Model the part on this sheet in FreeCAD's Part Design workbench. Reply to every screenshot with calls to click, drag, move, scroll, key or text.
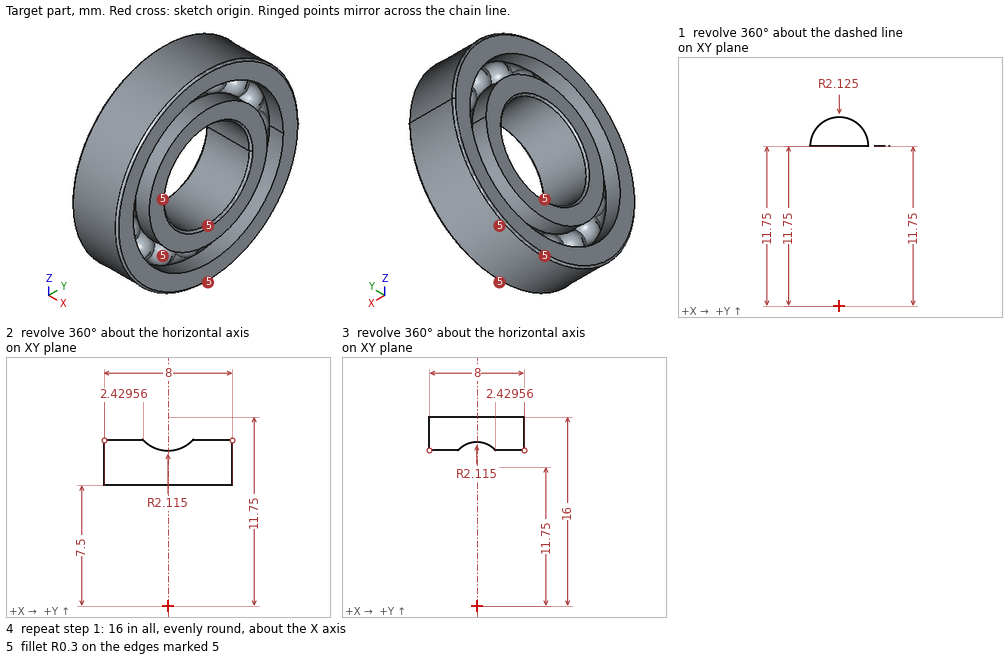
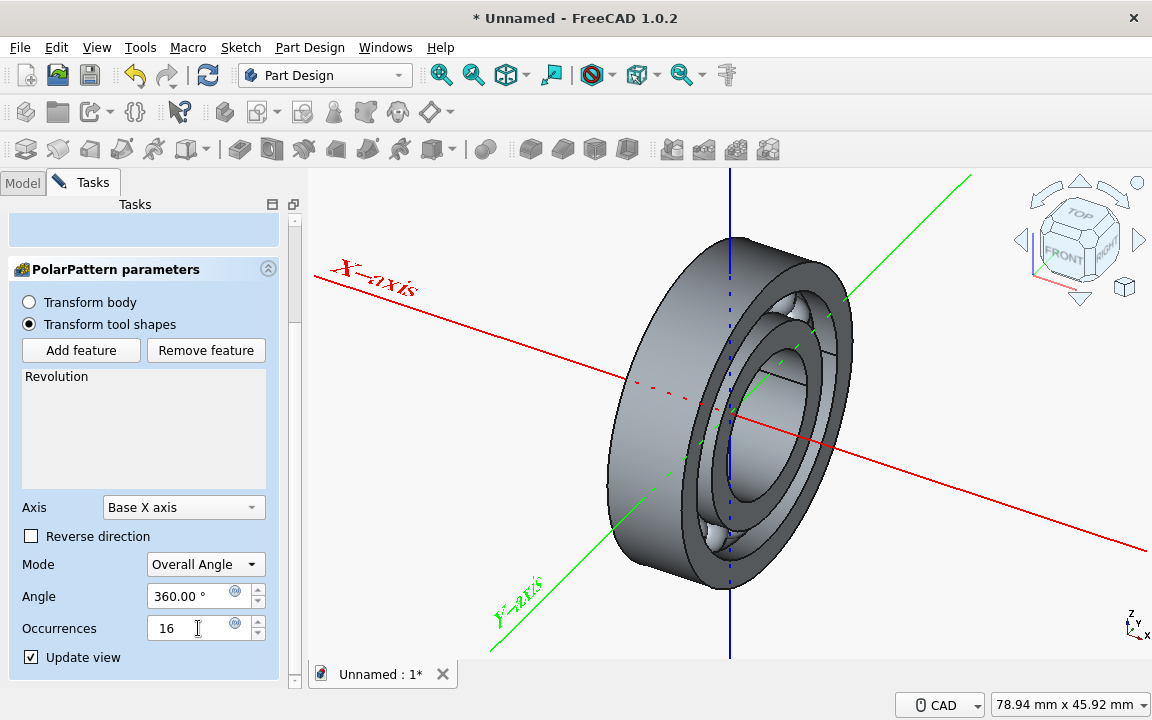
scroll(295, 451, up, 3)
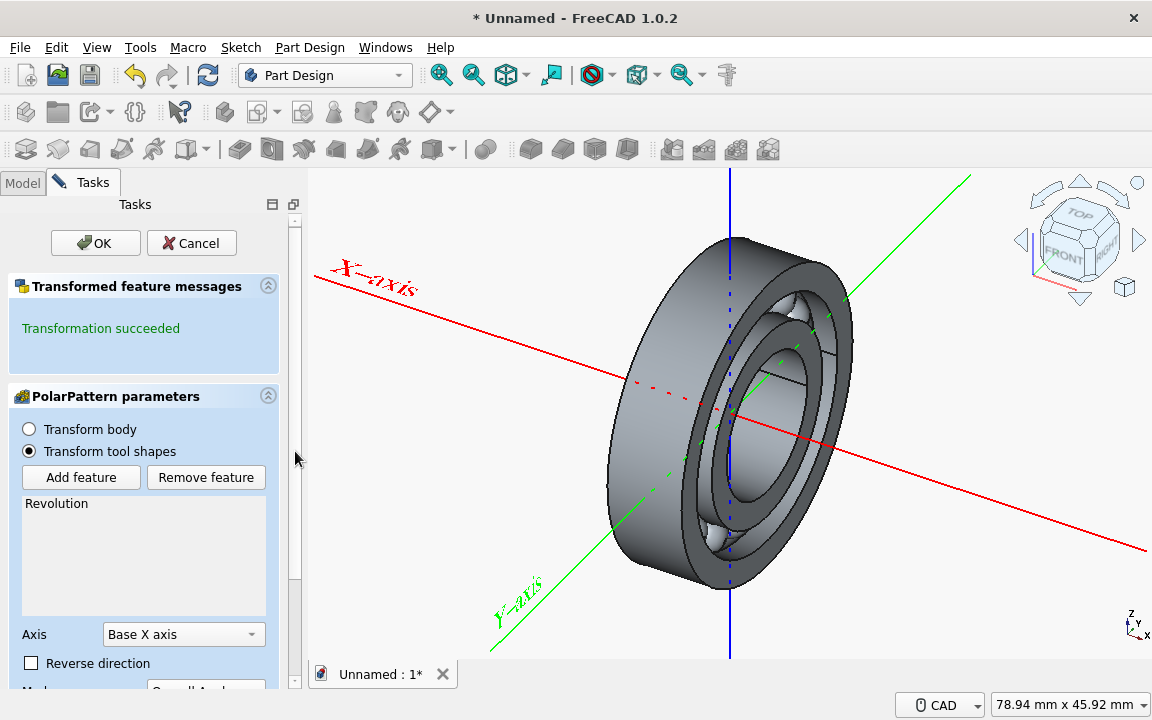
click(96, 243)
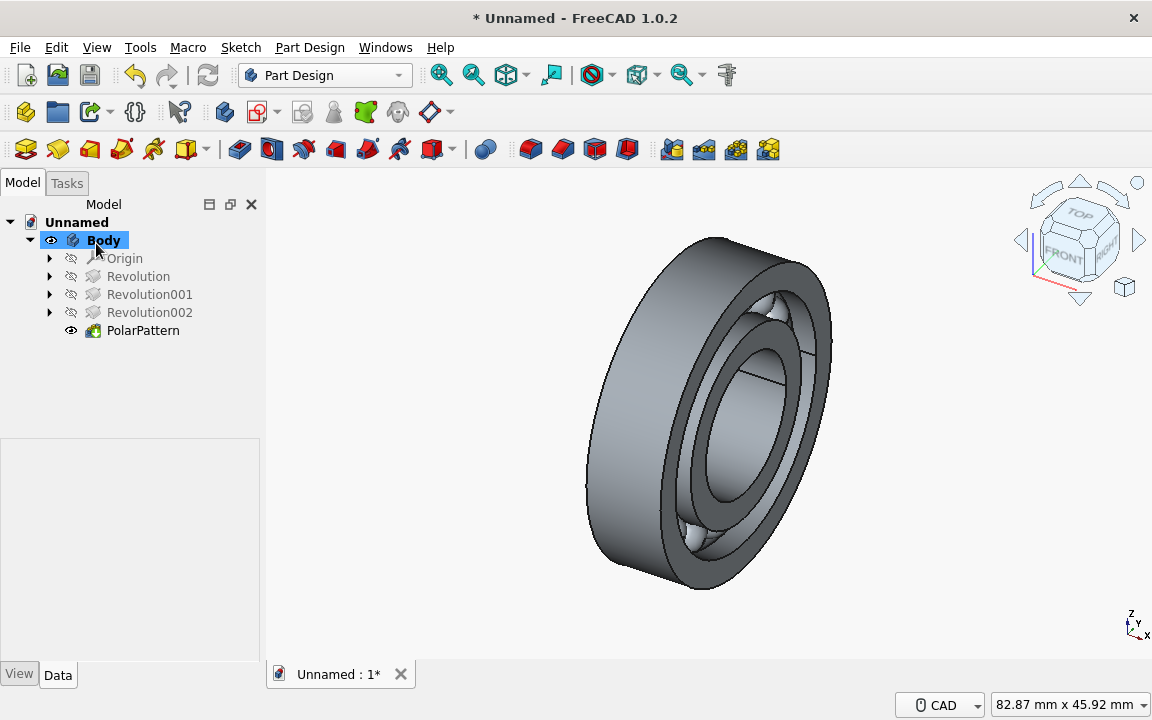
click(661, 510)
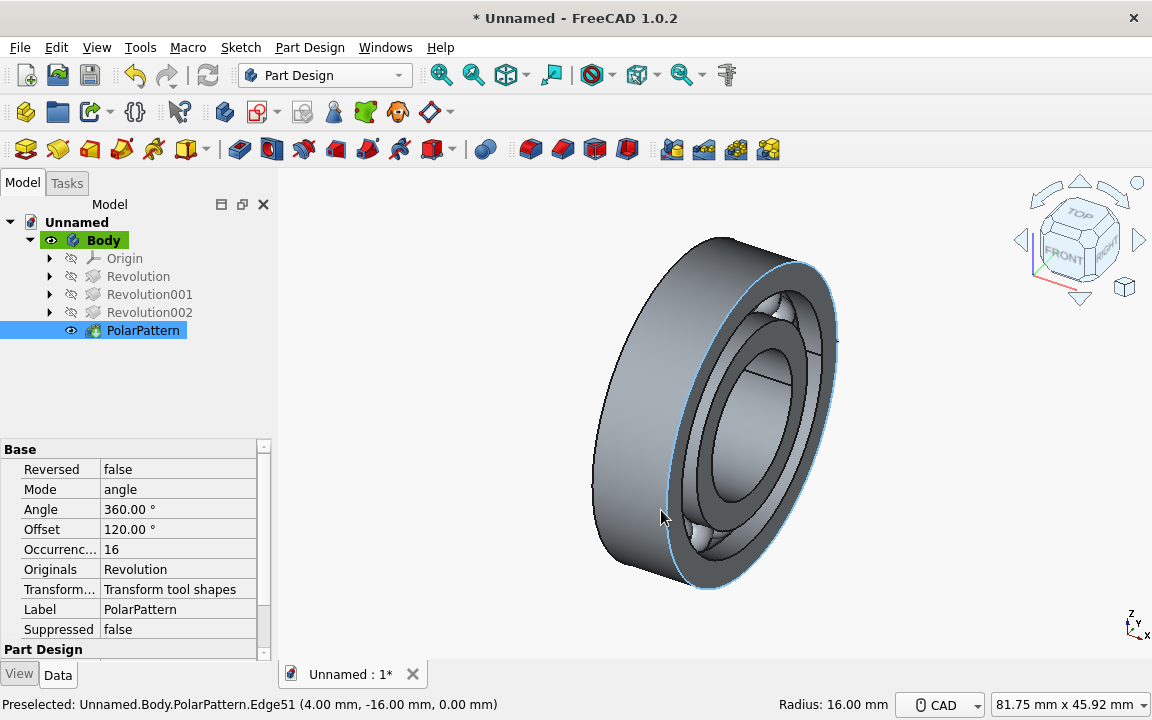
click(740, 500, ctrl)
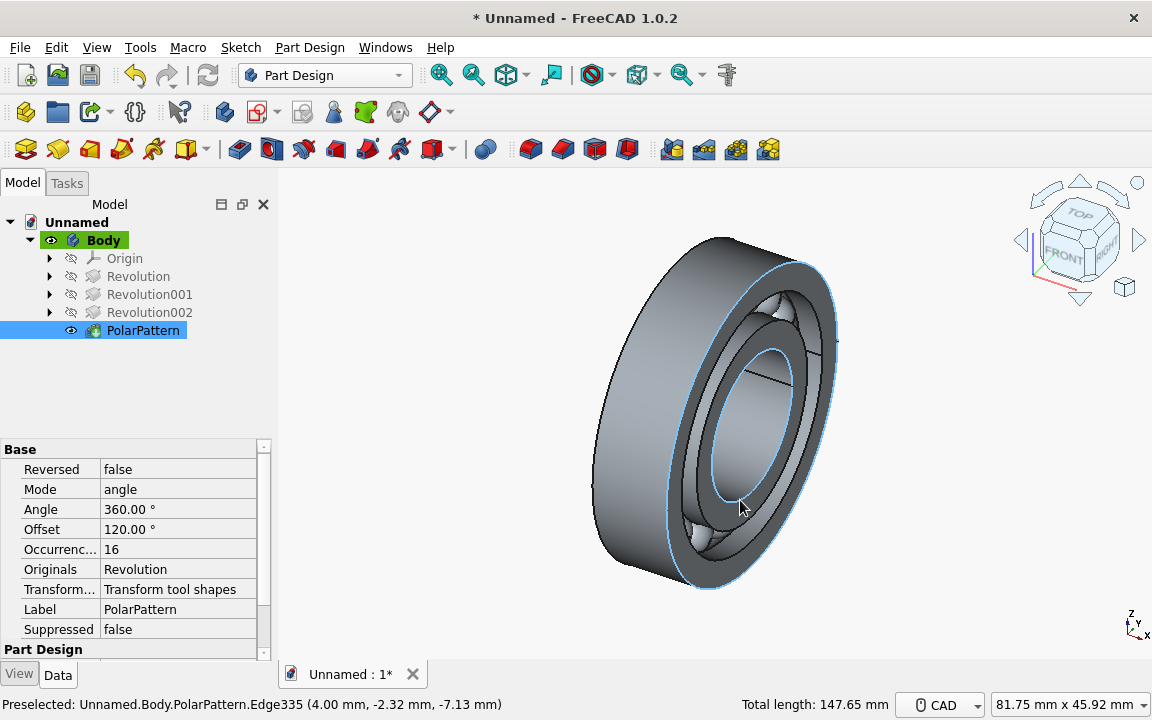
key(0)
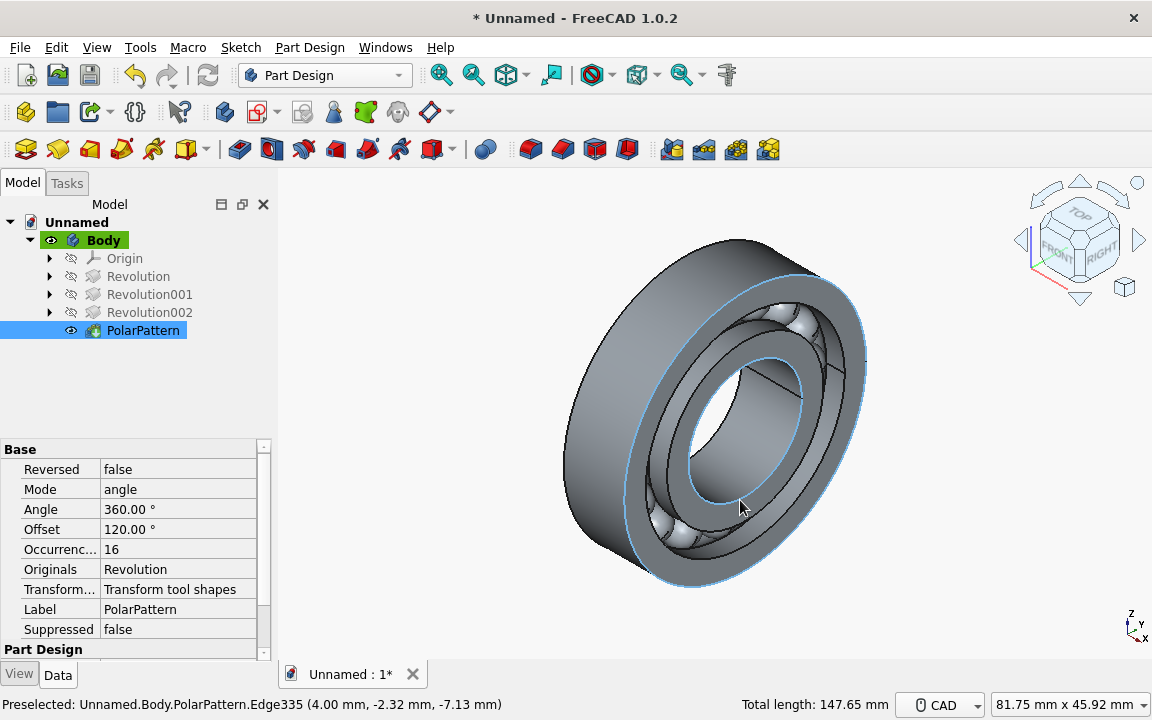
key(2)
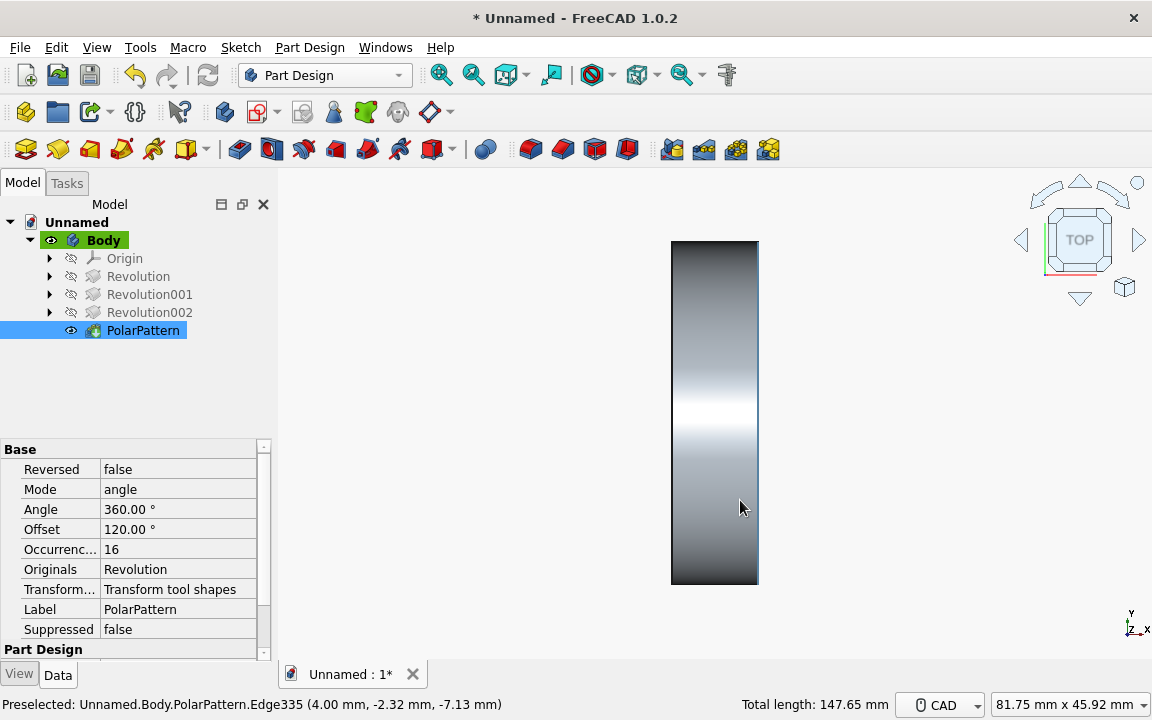
click(672, 551, ctrl)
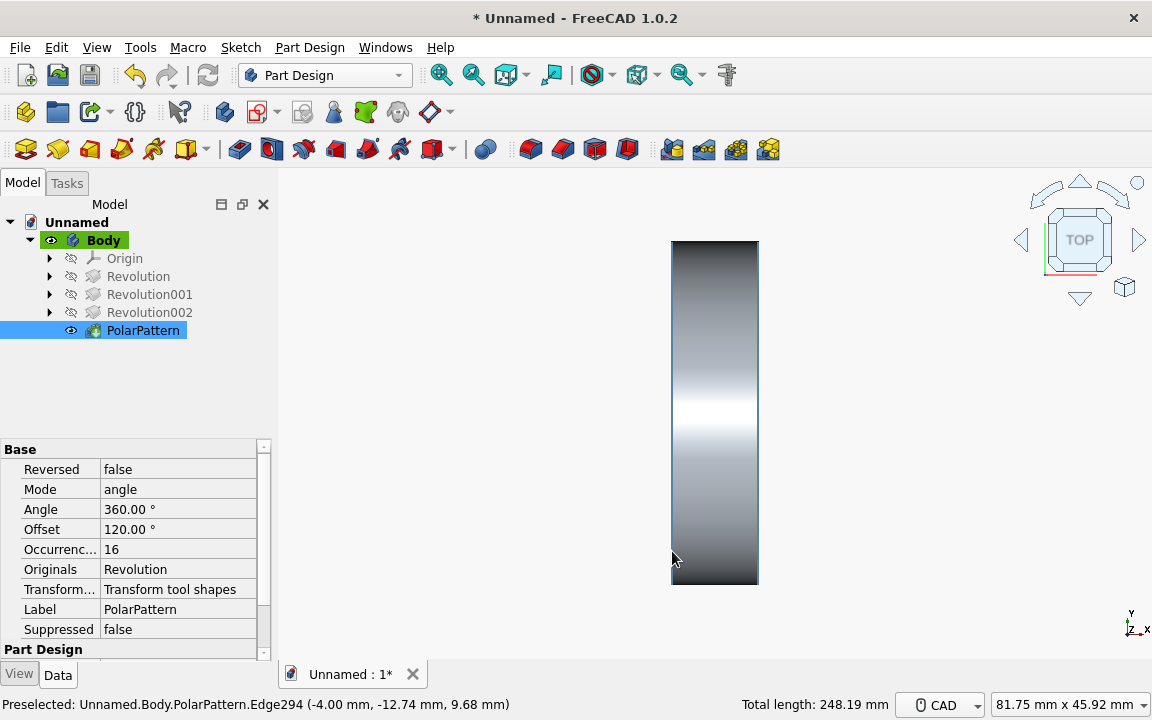
key(1)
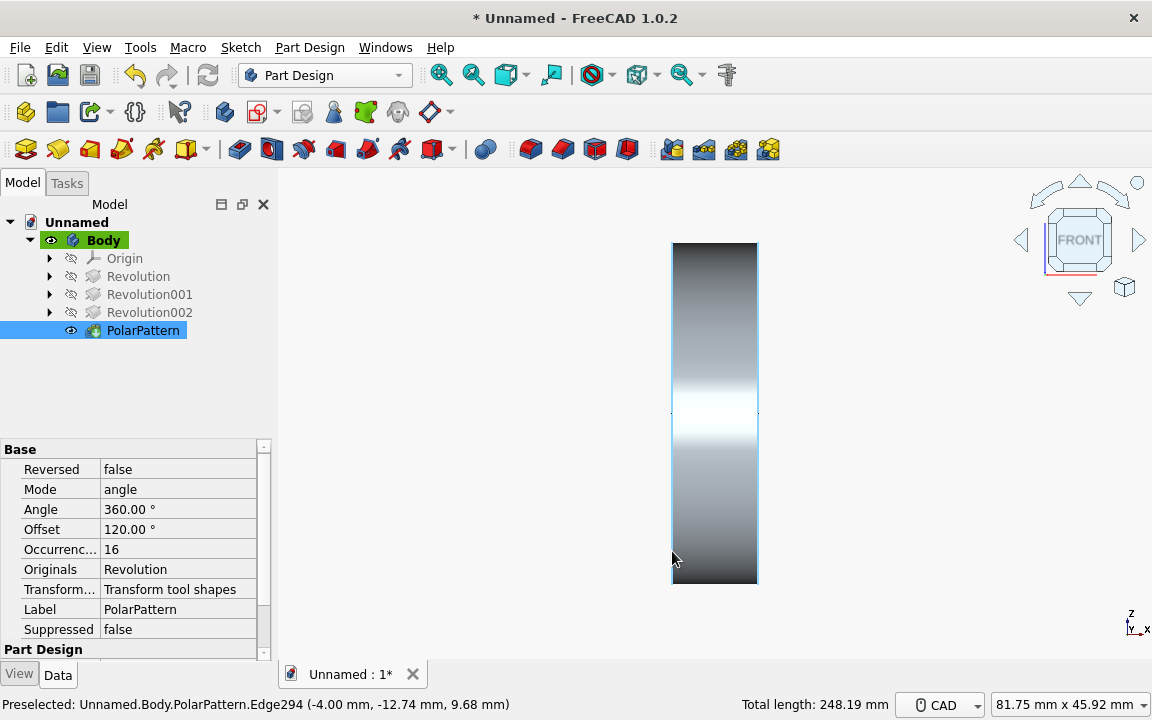
key(3)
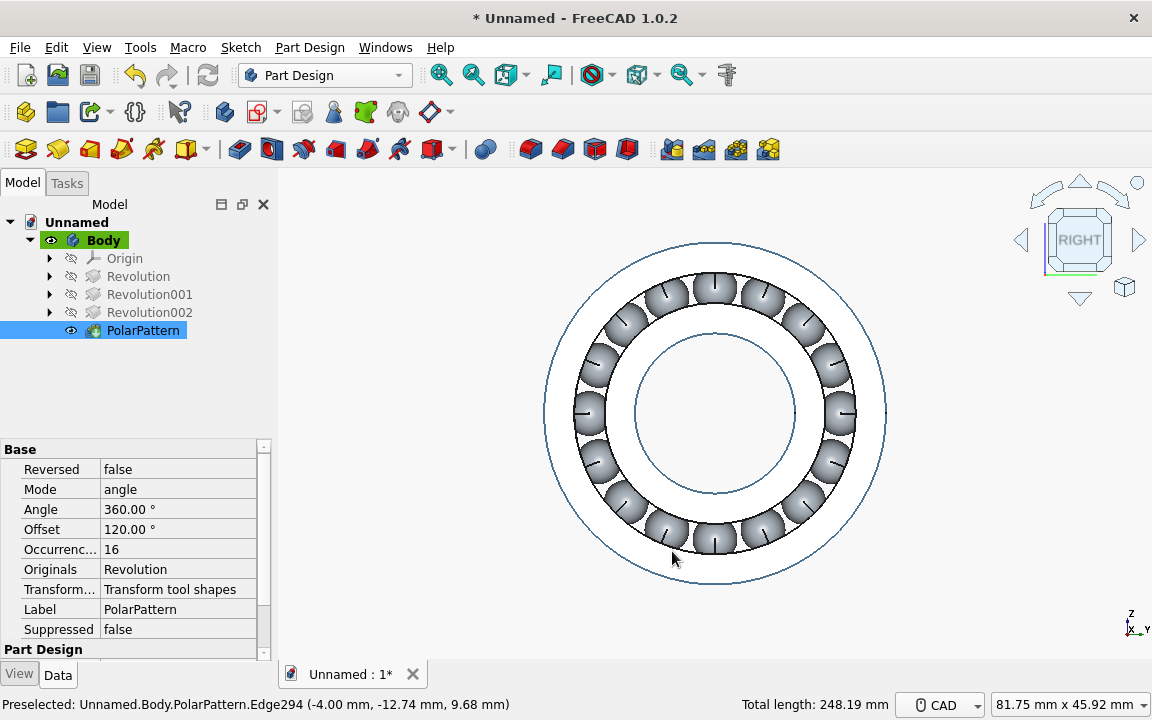
key(5)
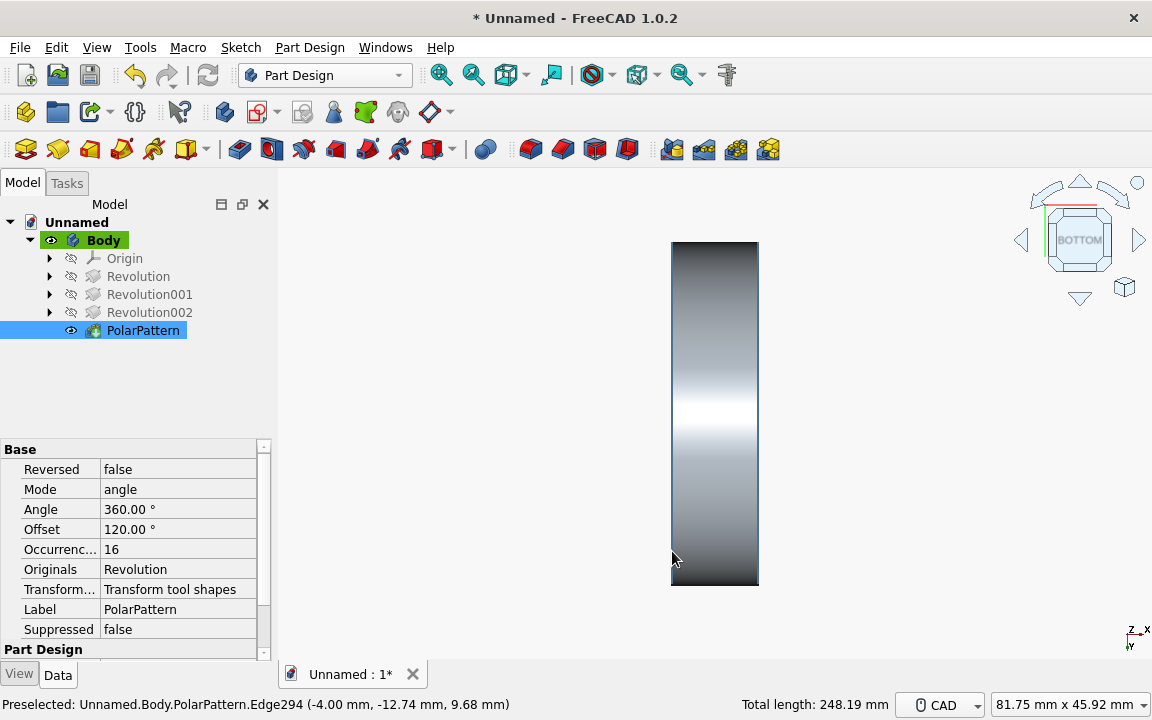
key(4)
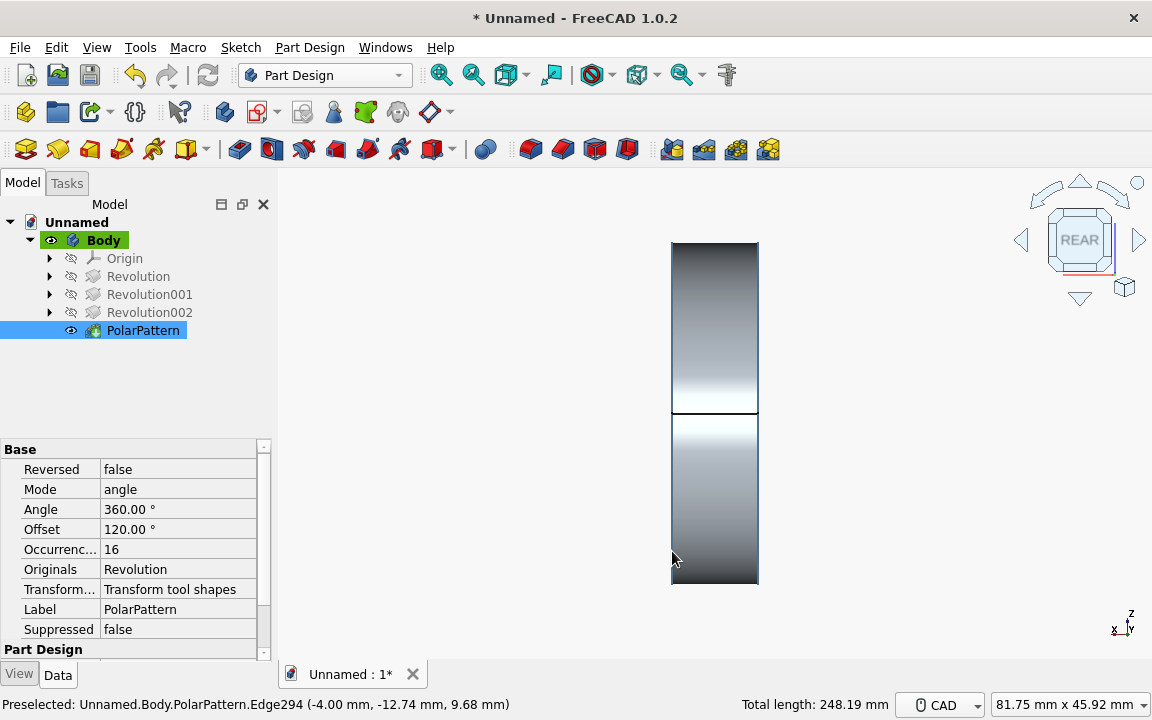
key(6)